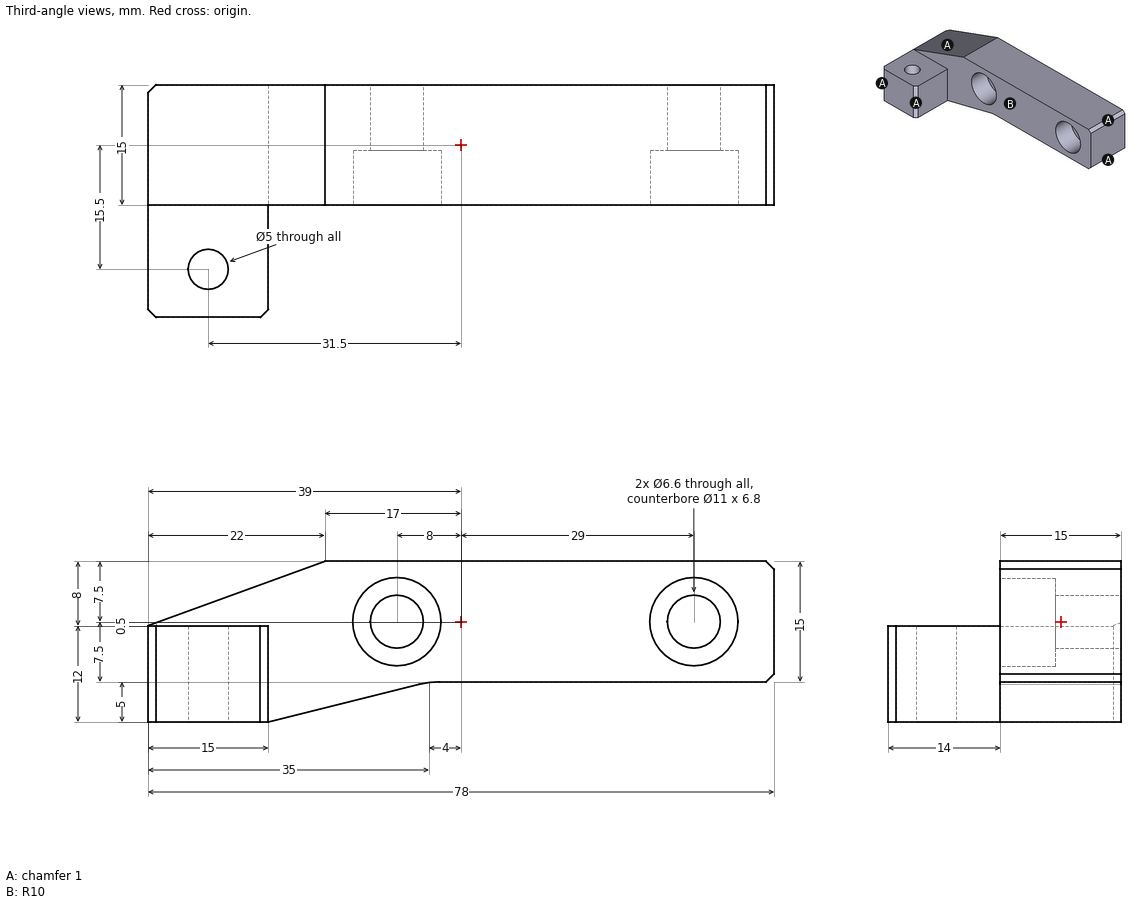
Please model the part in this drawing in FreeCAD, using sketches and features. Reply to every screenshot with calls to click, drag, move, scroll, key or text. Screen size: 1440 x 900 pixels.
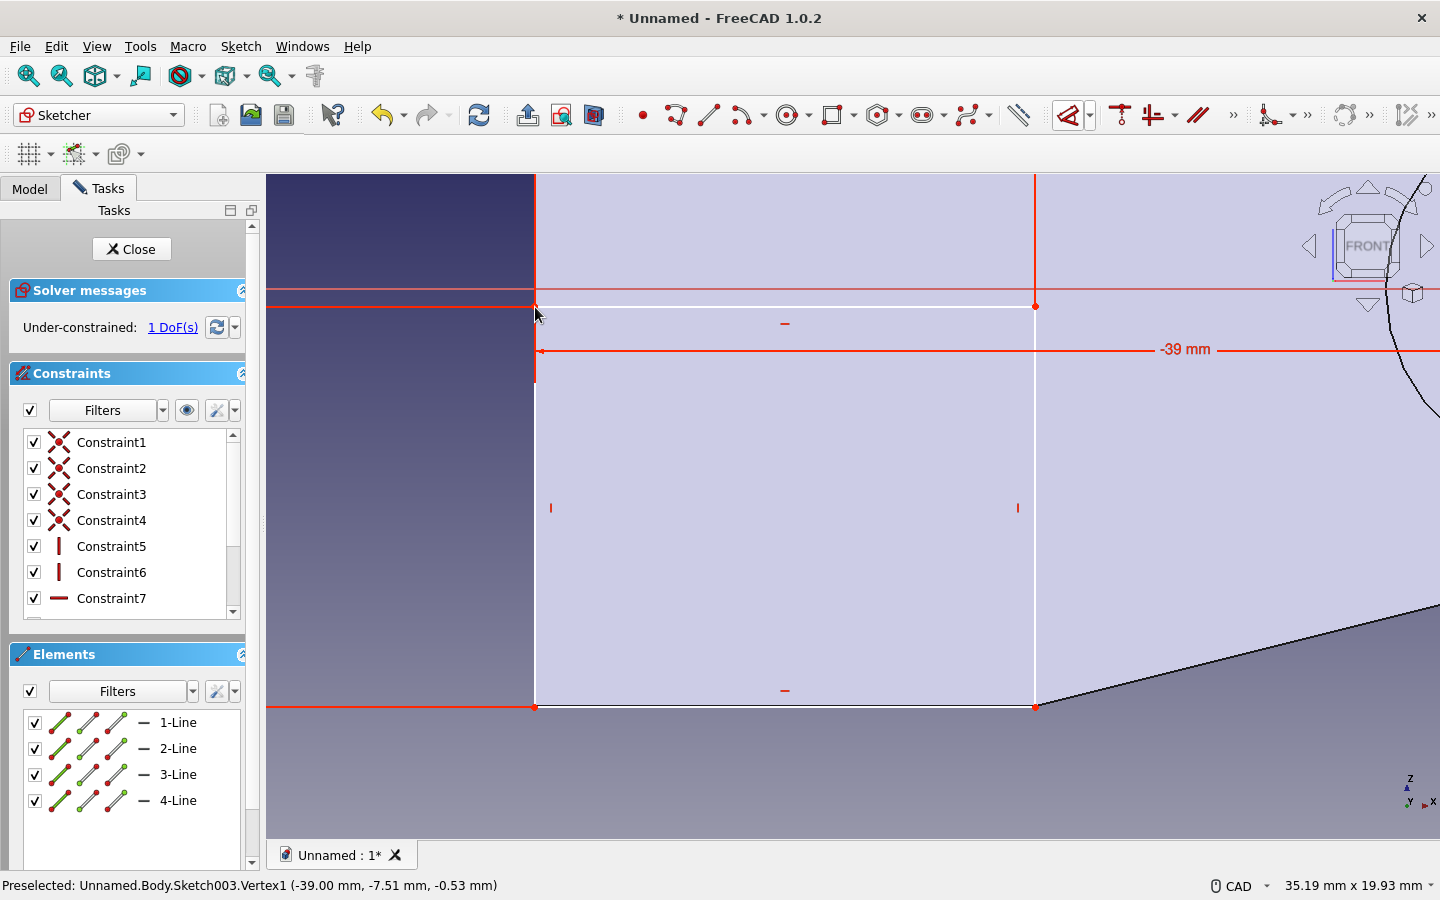
scroll(535, 307, up, 5)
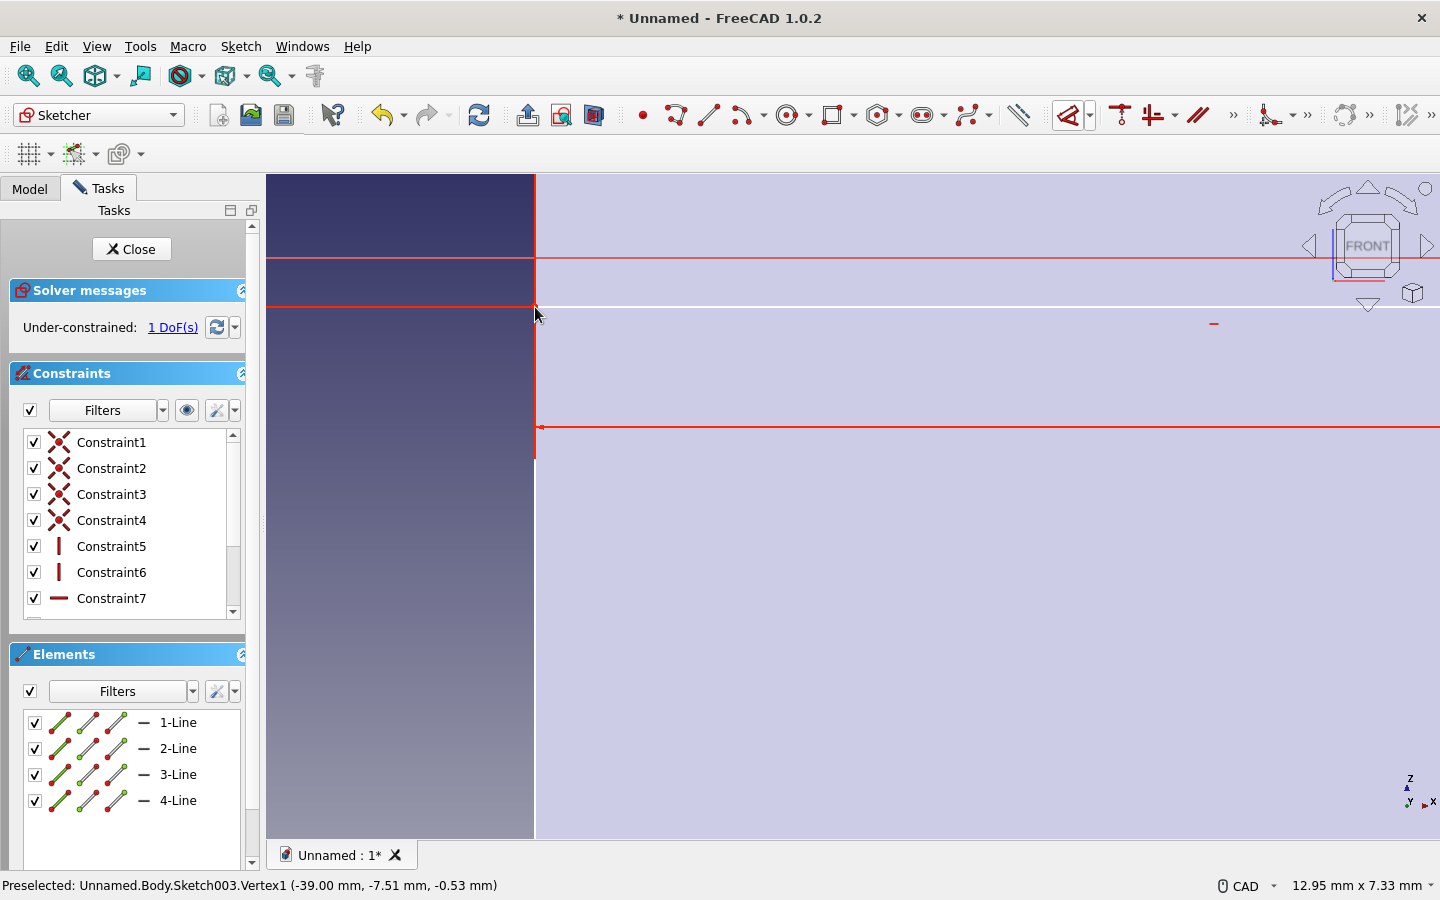
click(535, 307)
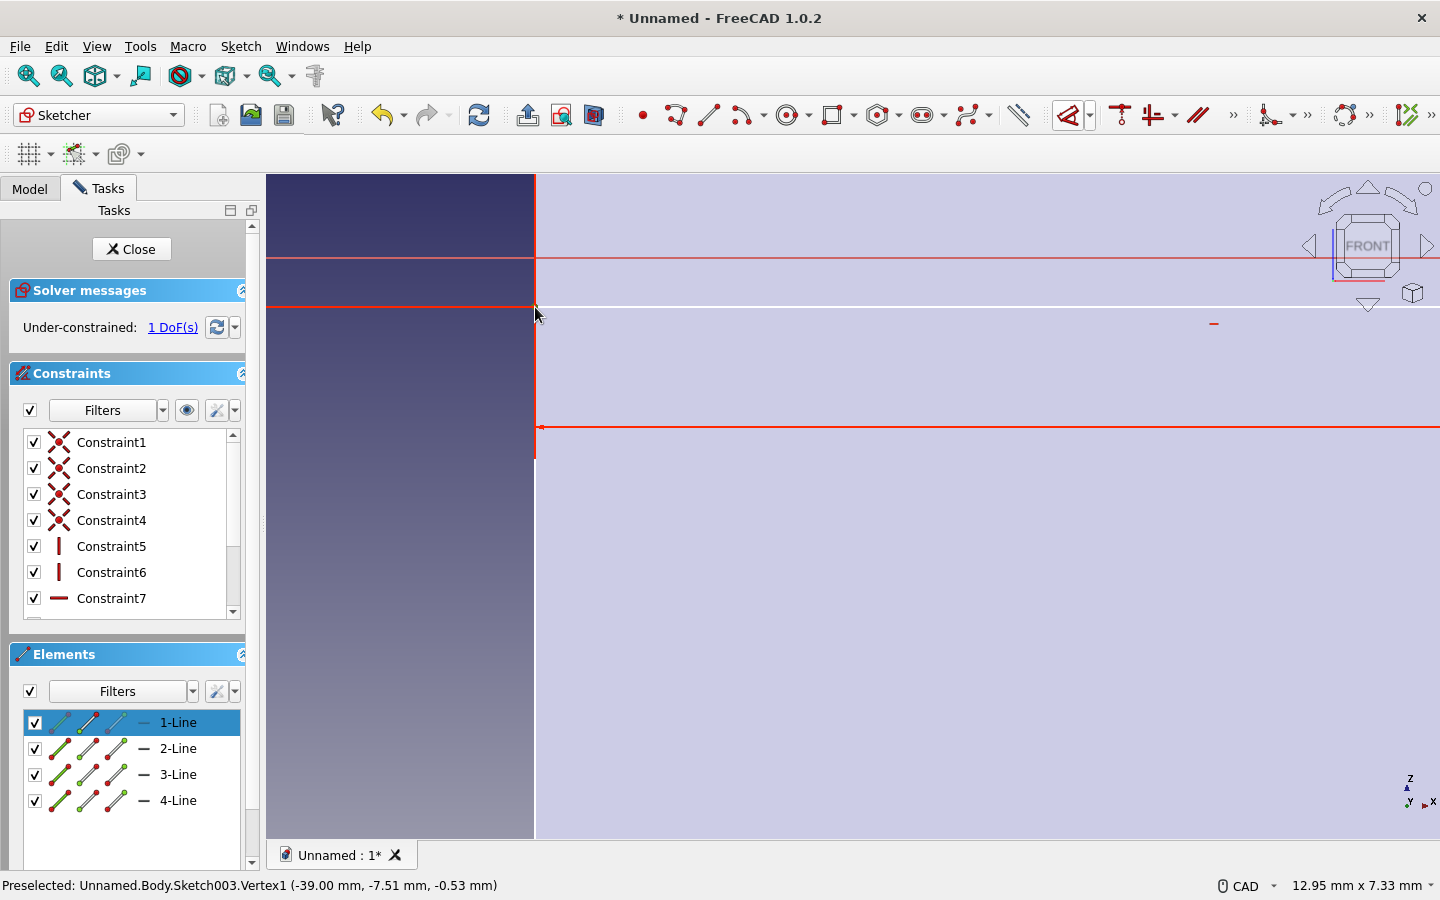
key(i)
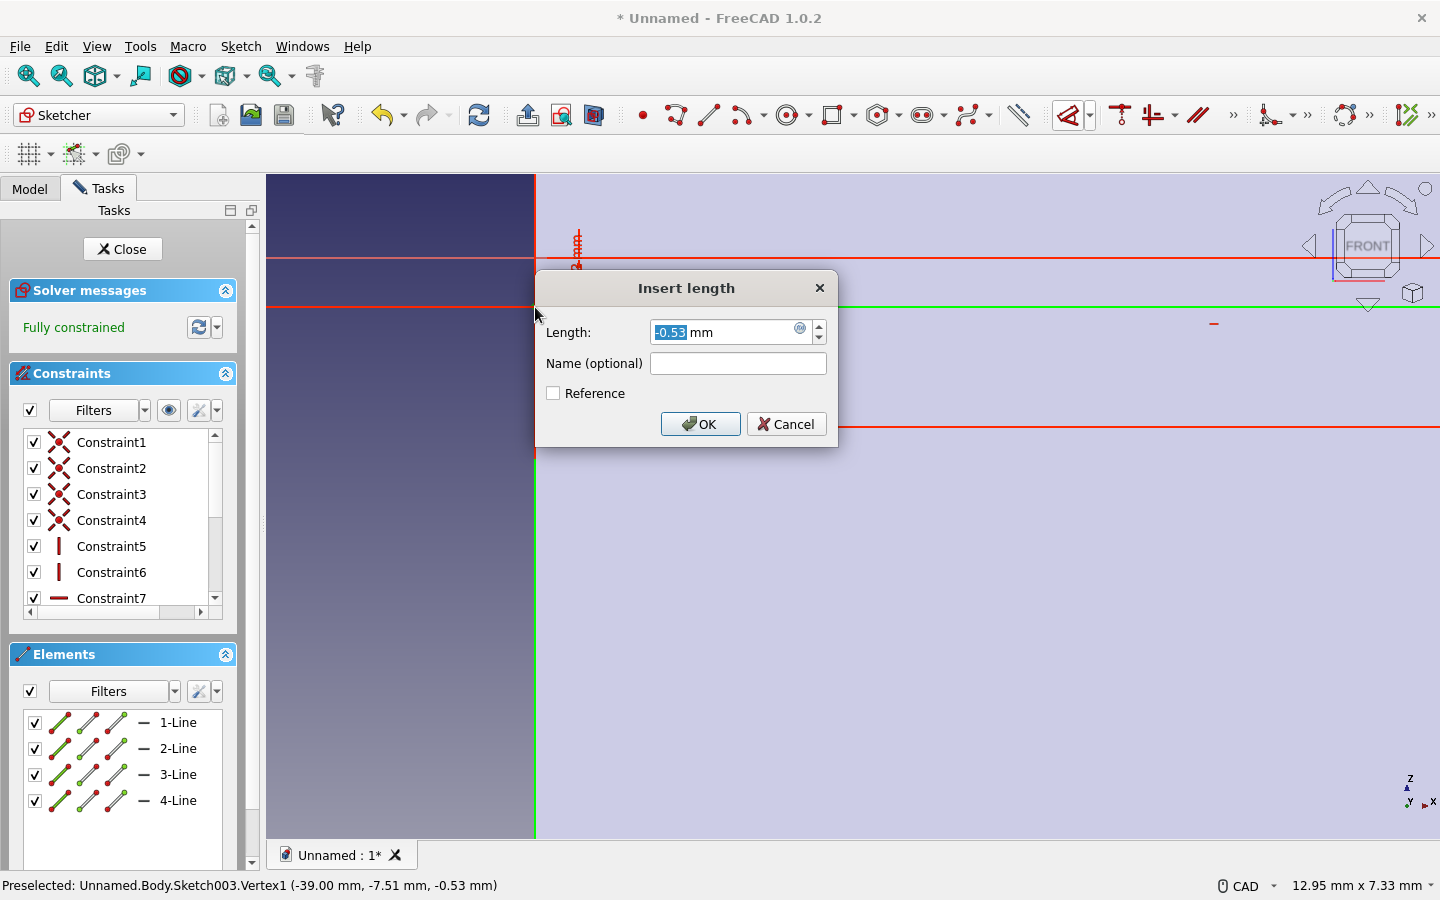
text(-0.5)
key(Return)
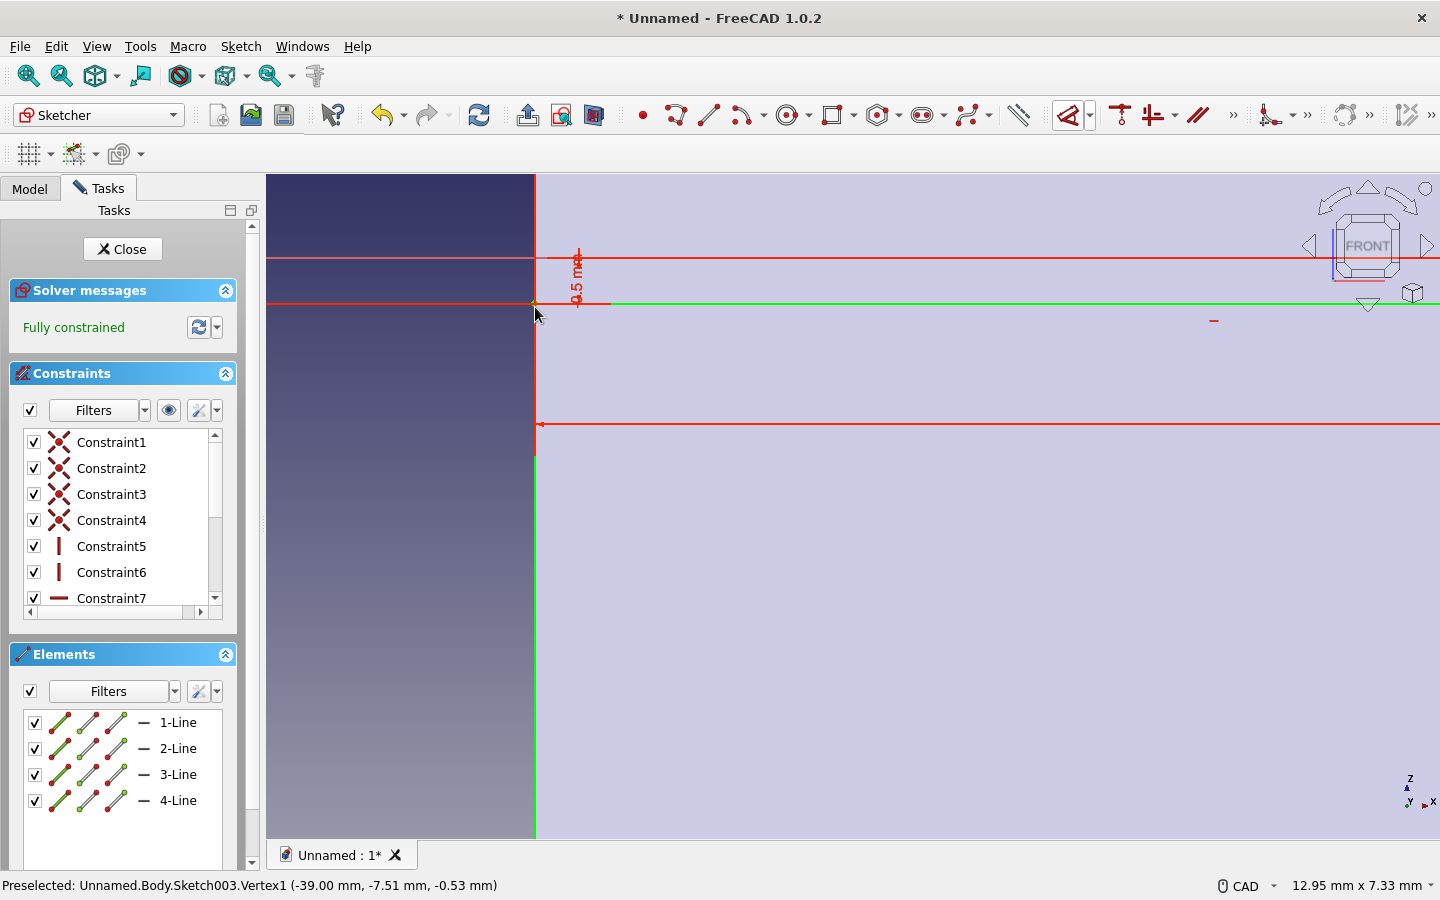
click(123, 249)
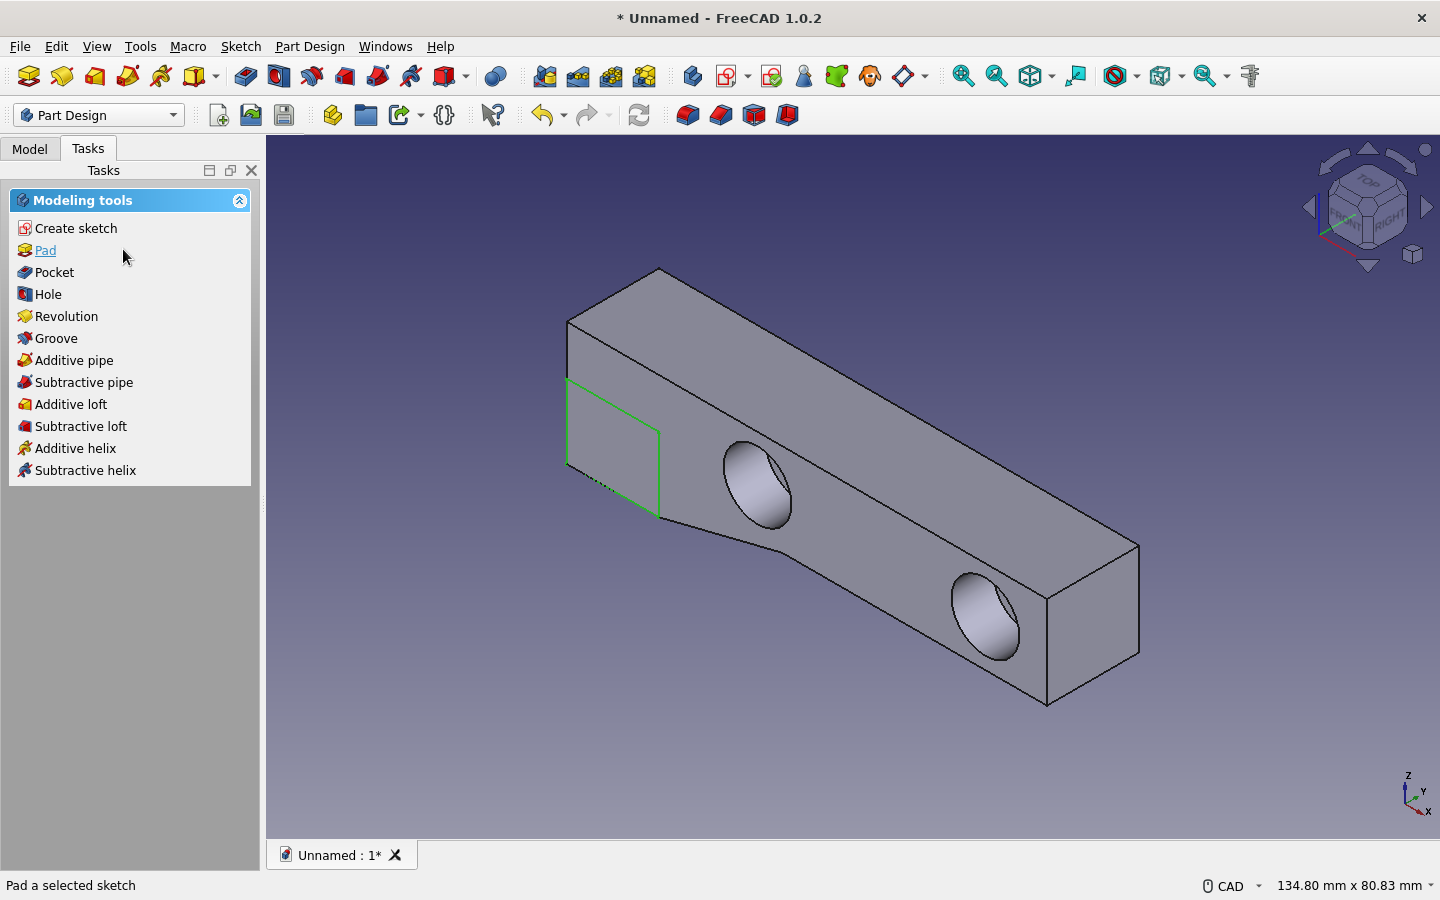
click(29, 76)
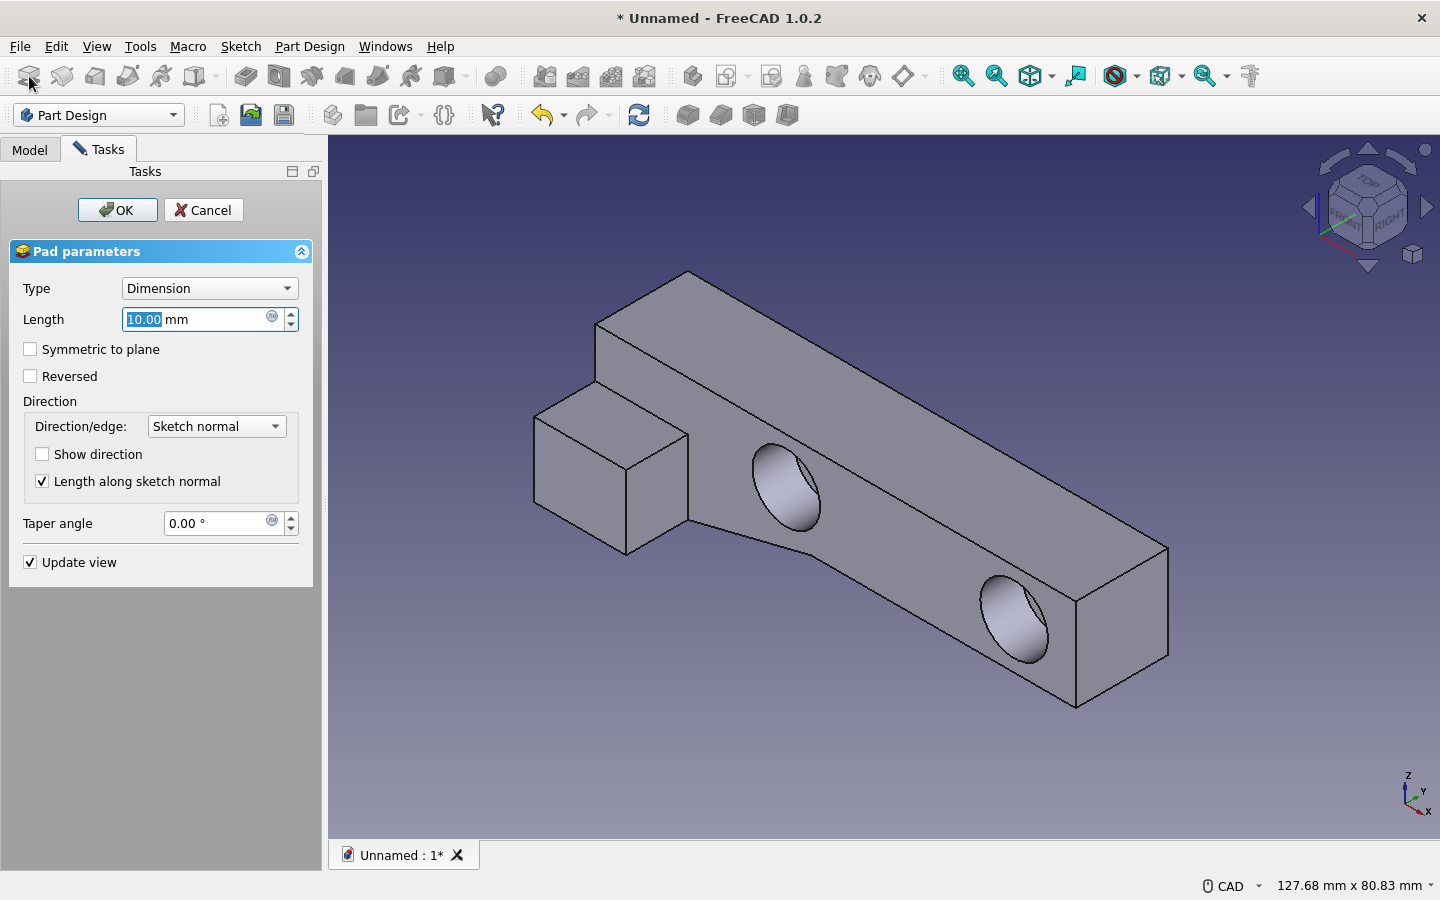
text(14)
key(Tab)